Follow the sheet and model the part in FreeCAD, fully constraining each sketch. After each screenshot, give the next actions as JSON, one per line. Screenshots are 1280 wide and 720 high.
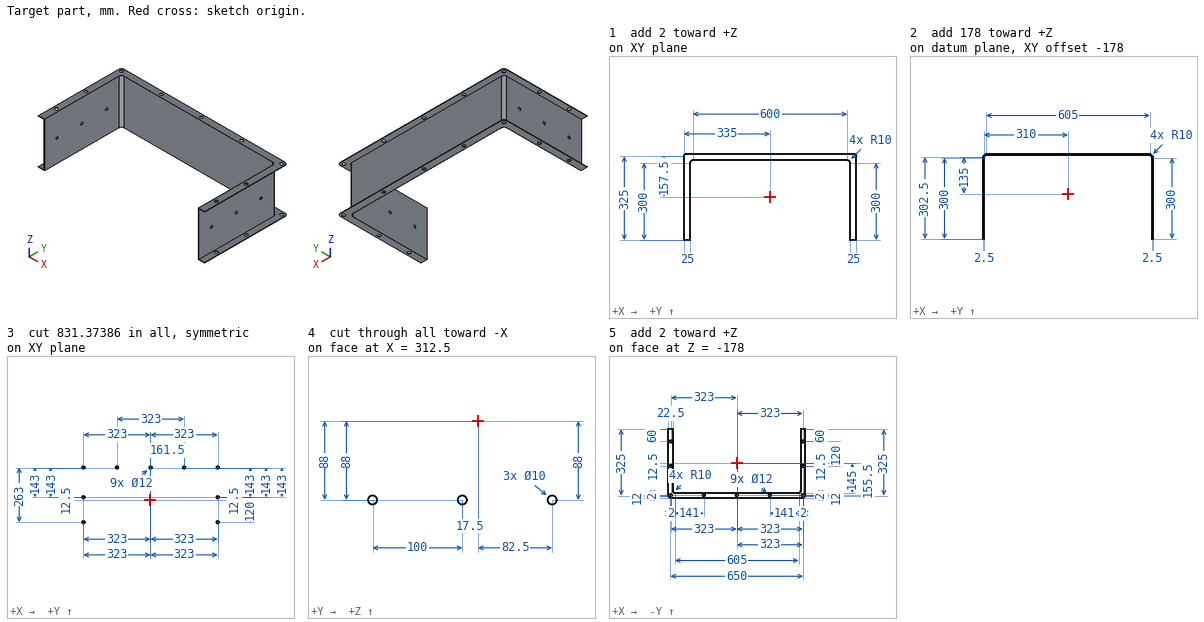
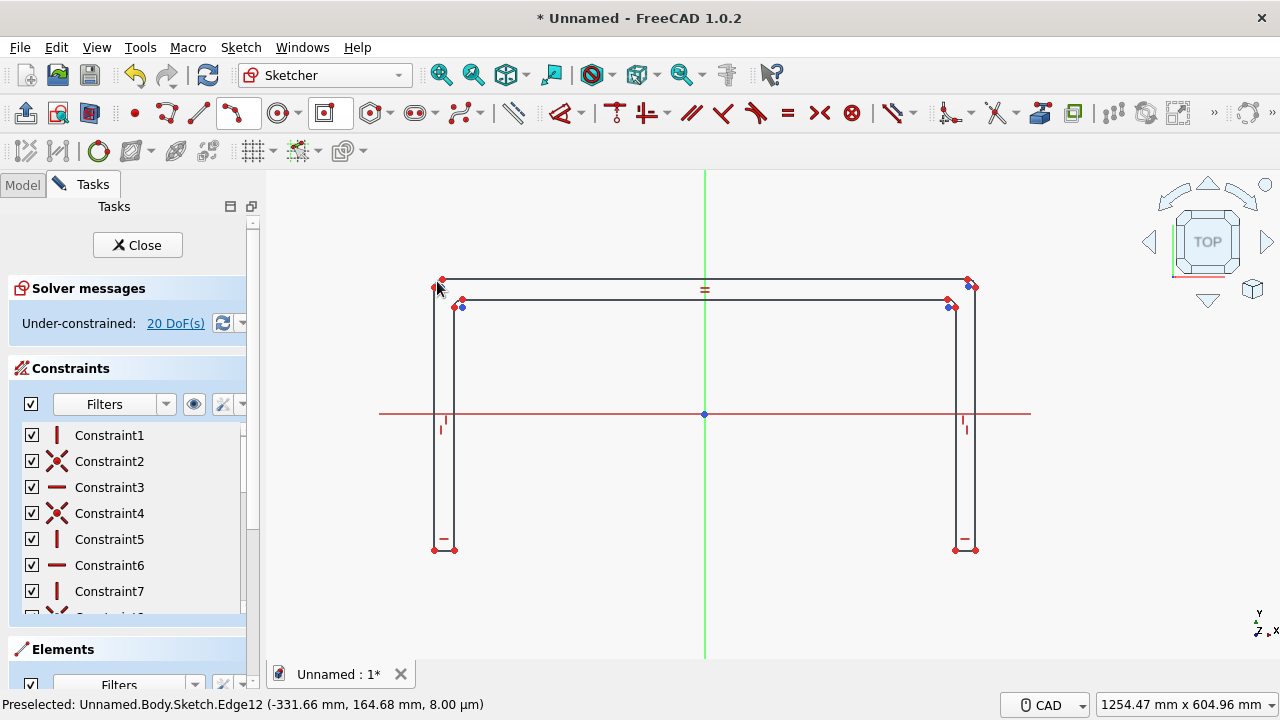
{"action": "left_click", "coordinate": [434, 367]}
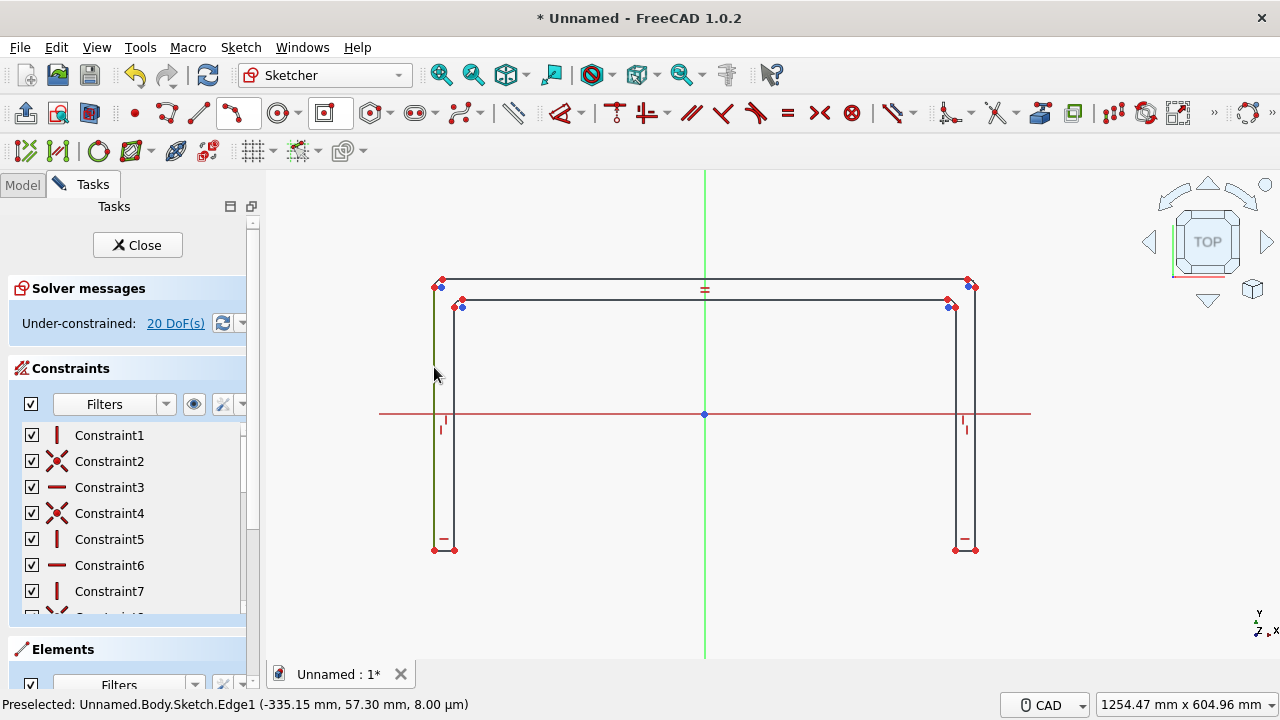
{"action": "scroll", "coordinate": [436, 282], "scroll_direction": "up", "scroll_amount": 4}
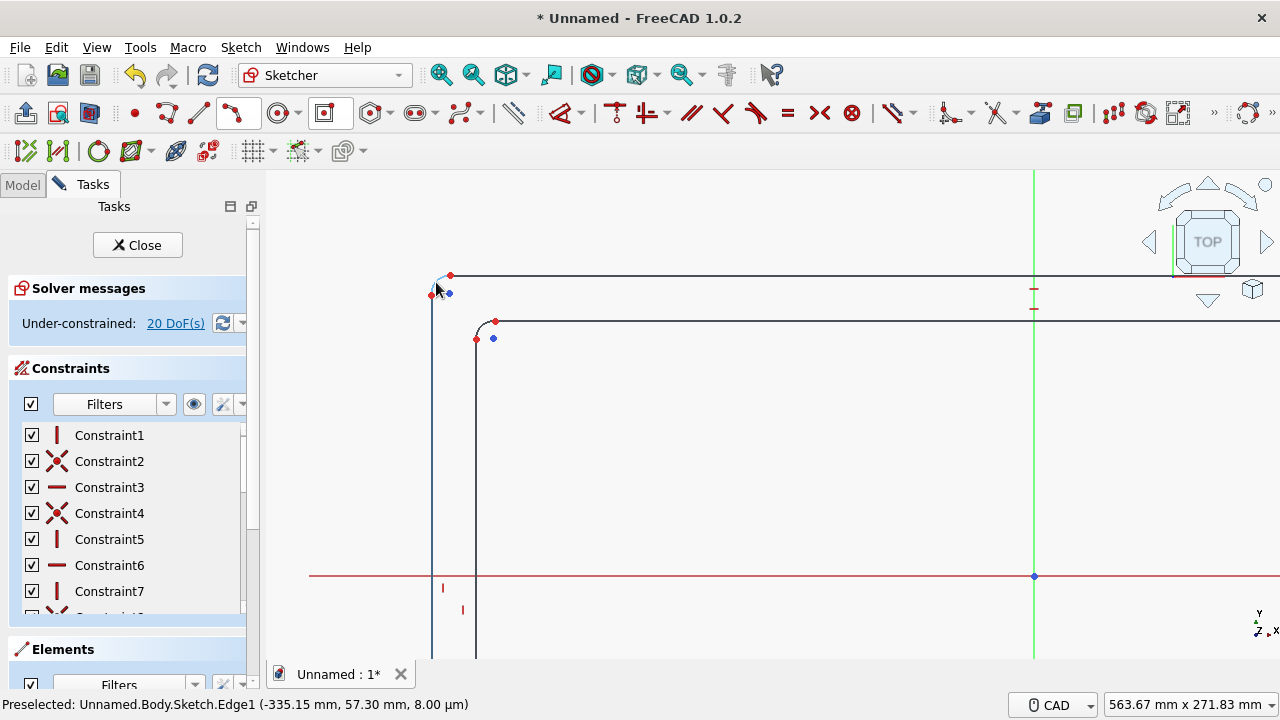
{"action": "left_click", "coordinate": [436, 281]}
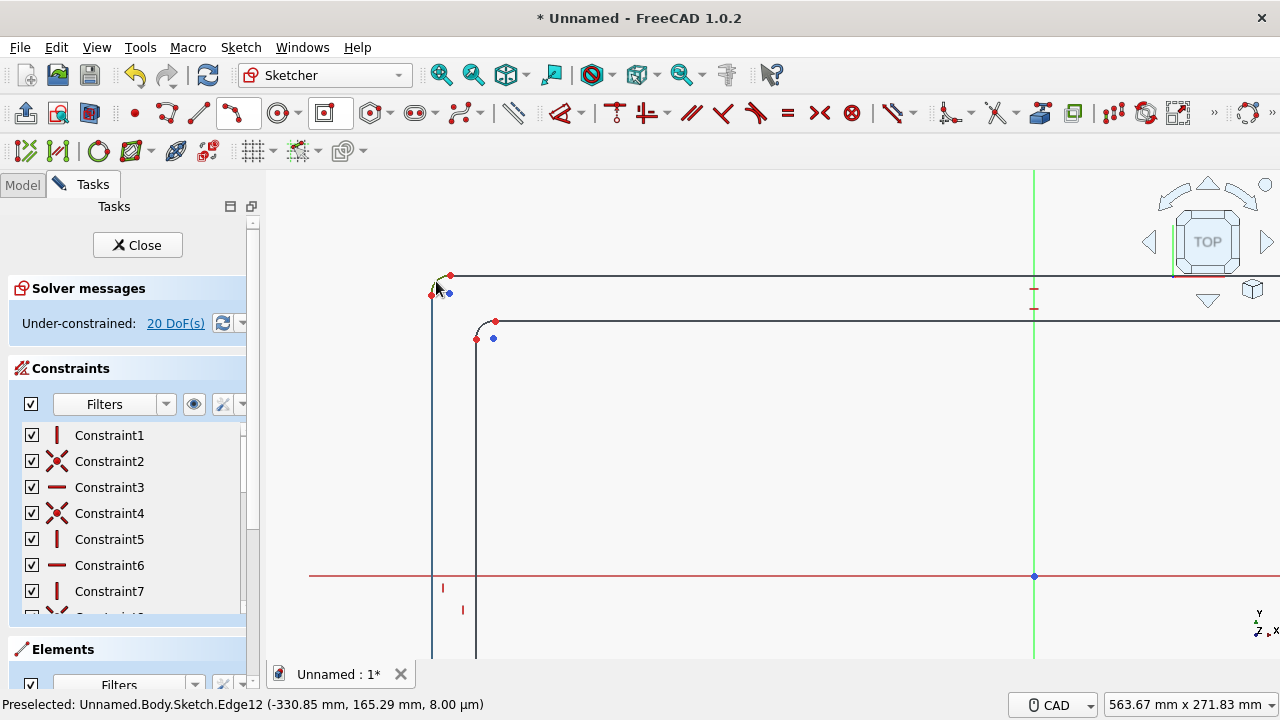
{"action": "left_click", "coordinate": [756, 114]}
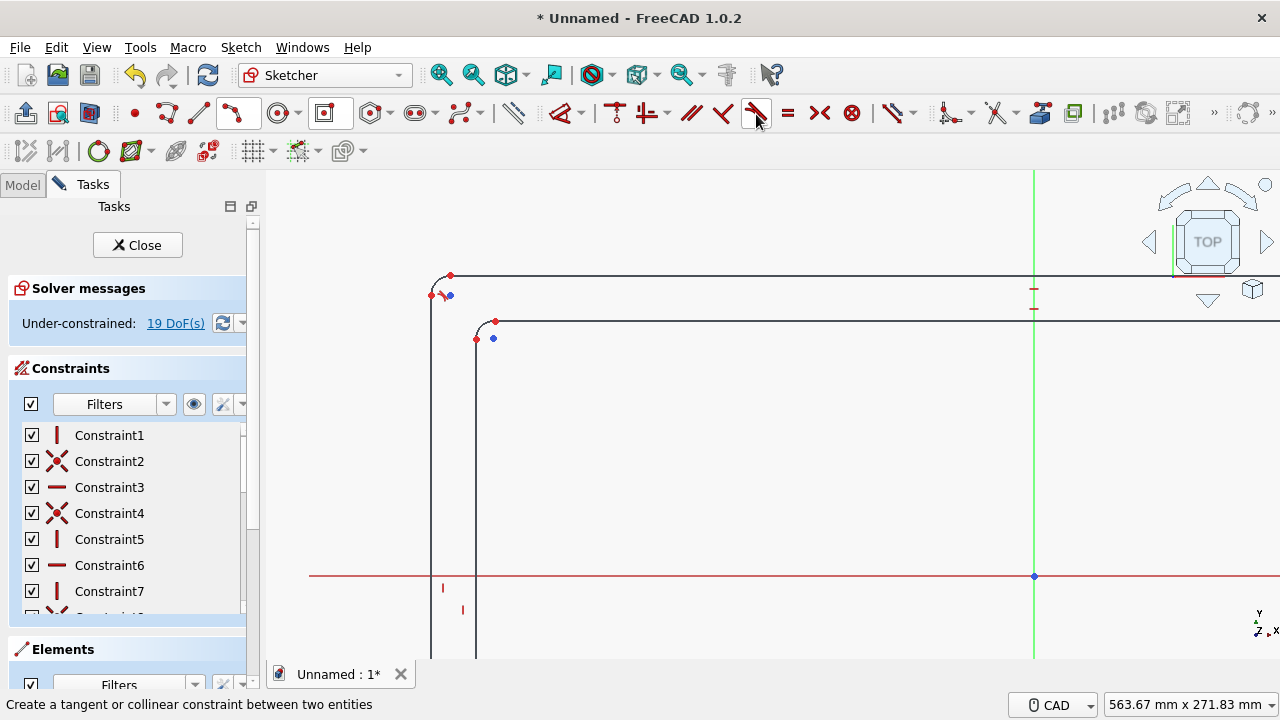
{"action": "left_click", "coordinate": [476, 502]}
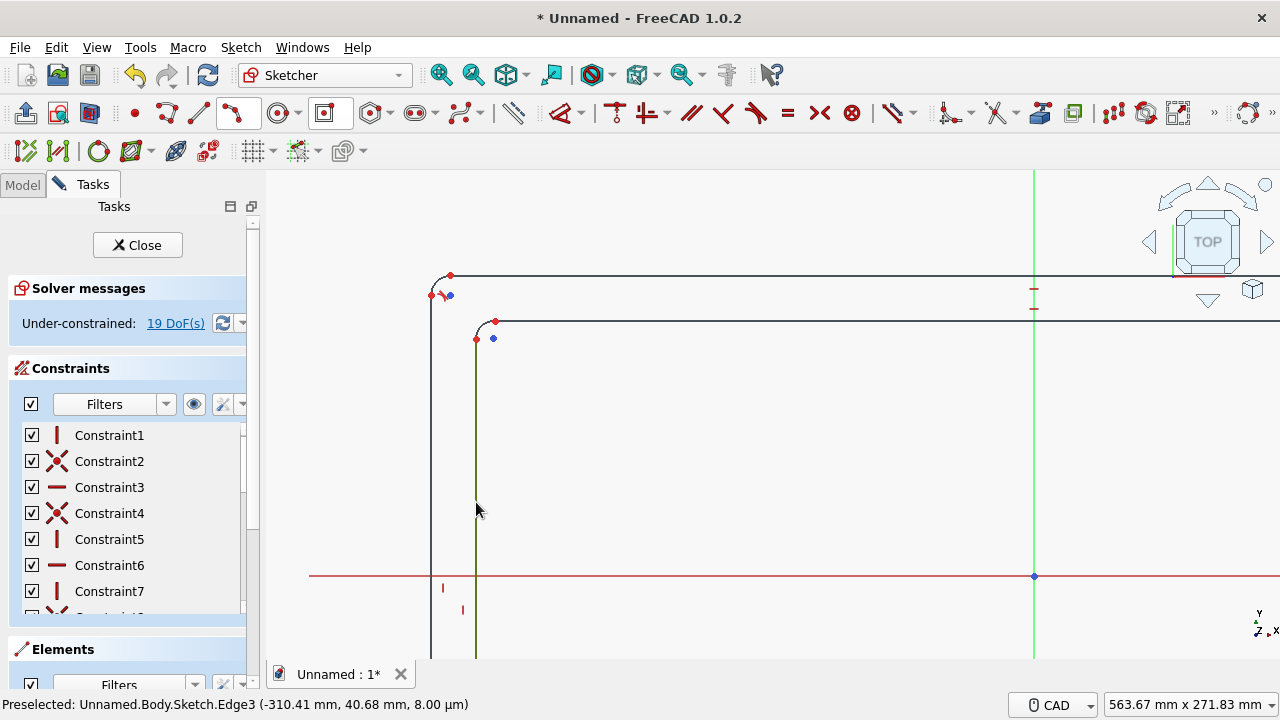
{"action": "left_click", "coordinate": [482, 326]}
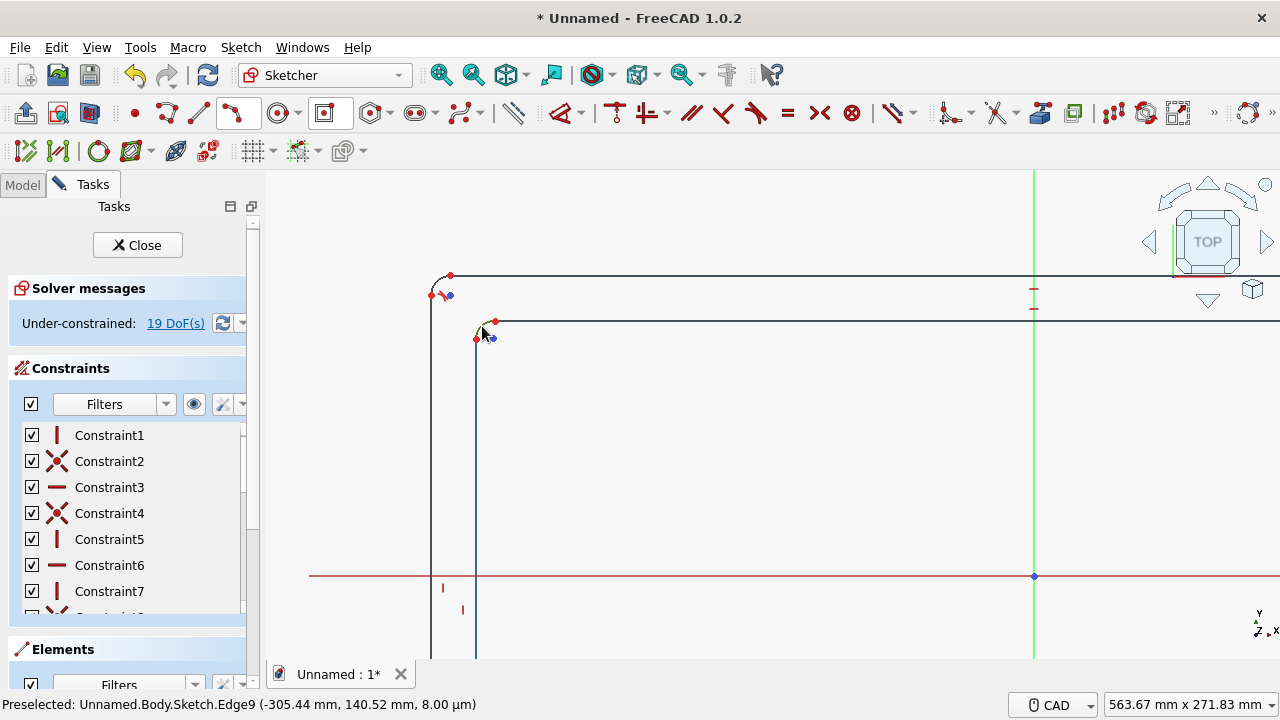
{"action": "left_click", "coordinate": [756, 114]}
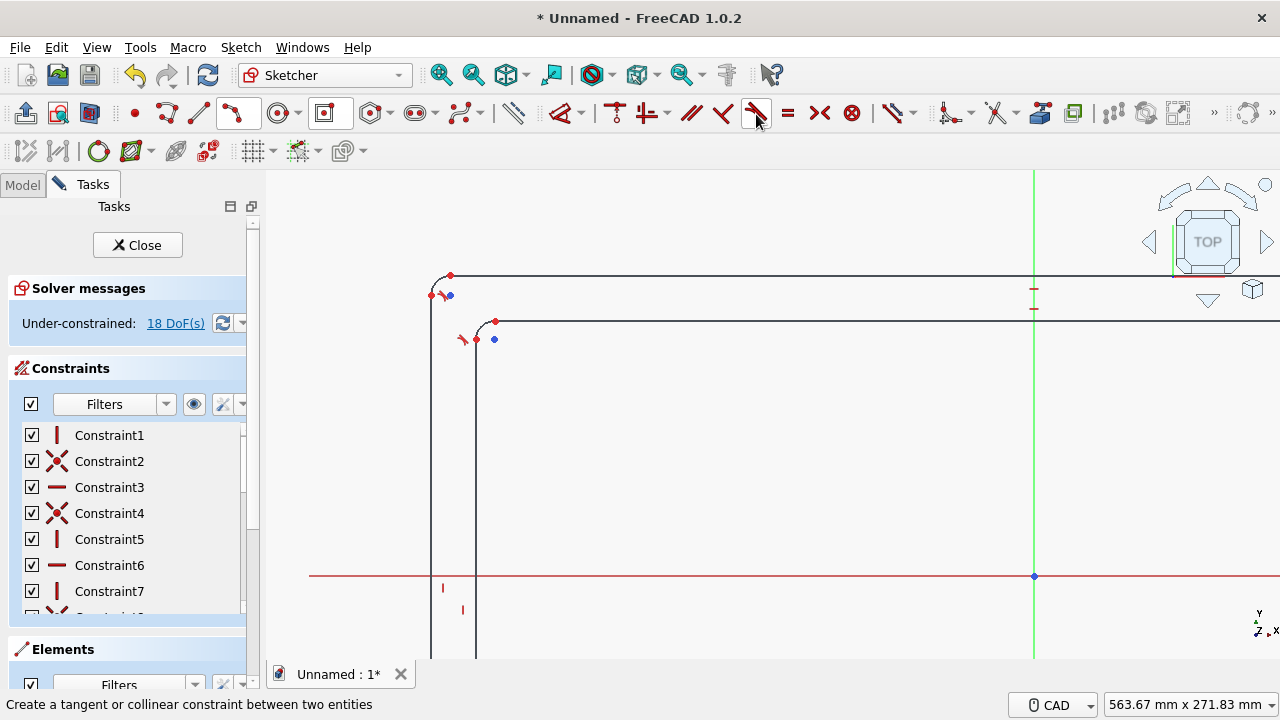
{"action": "left_click", "coordinate": [819, 321]}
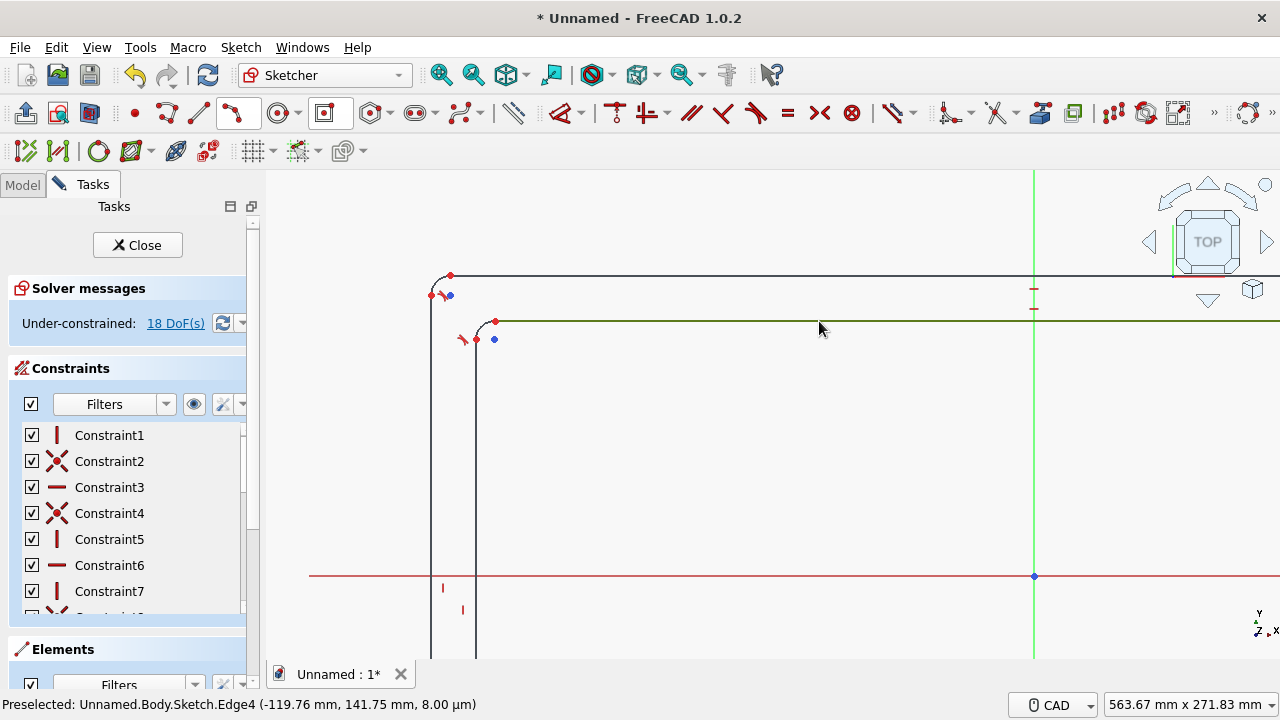
{"action": "left_click", "coordinate": [482, 326]}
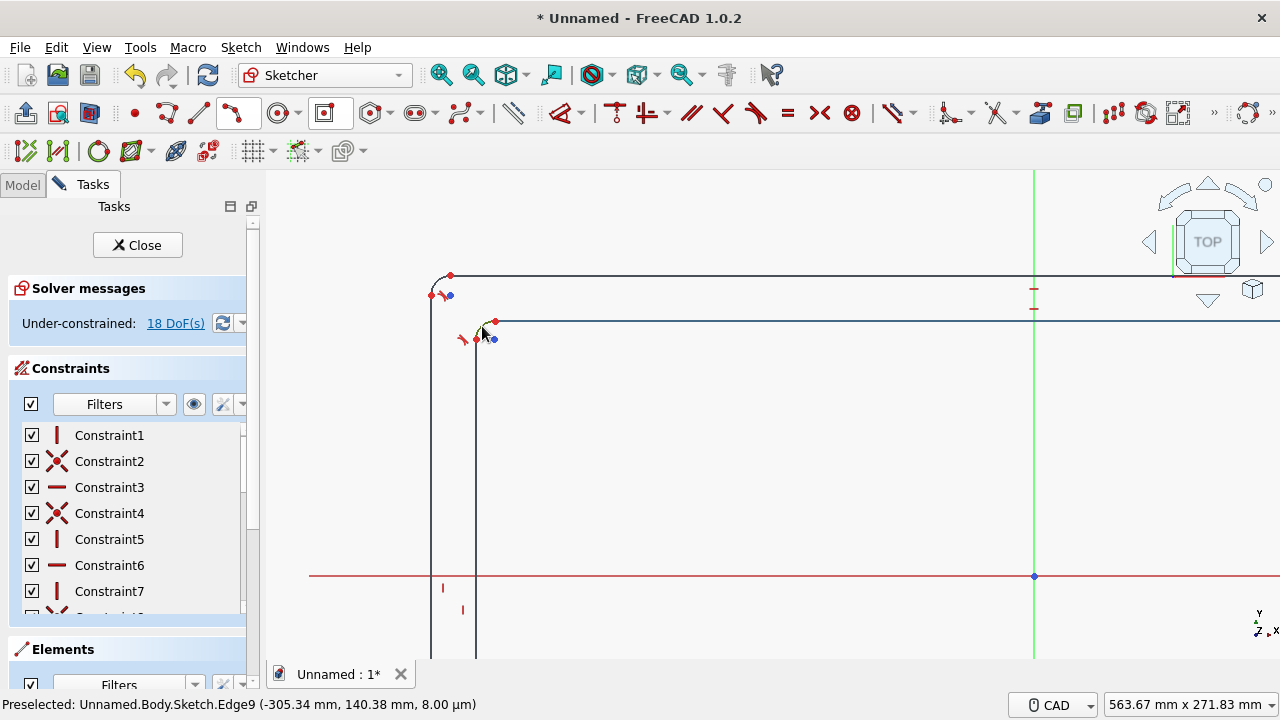
{"action": "key", "text": "t"}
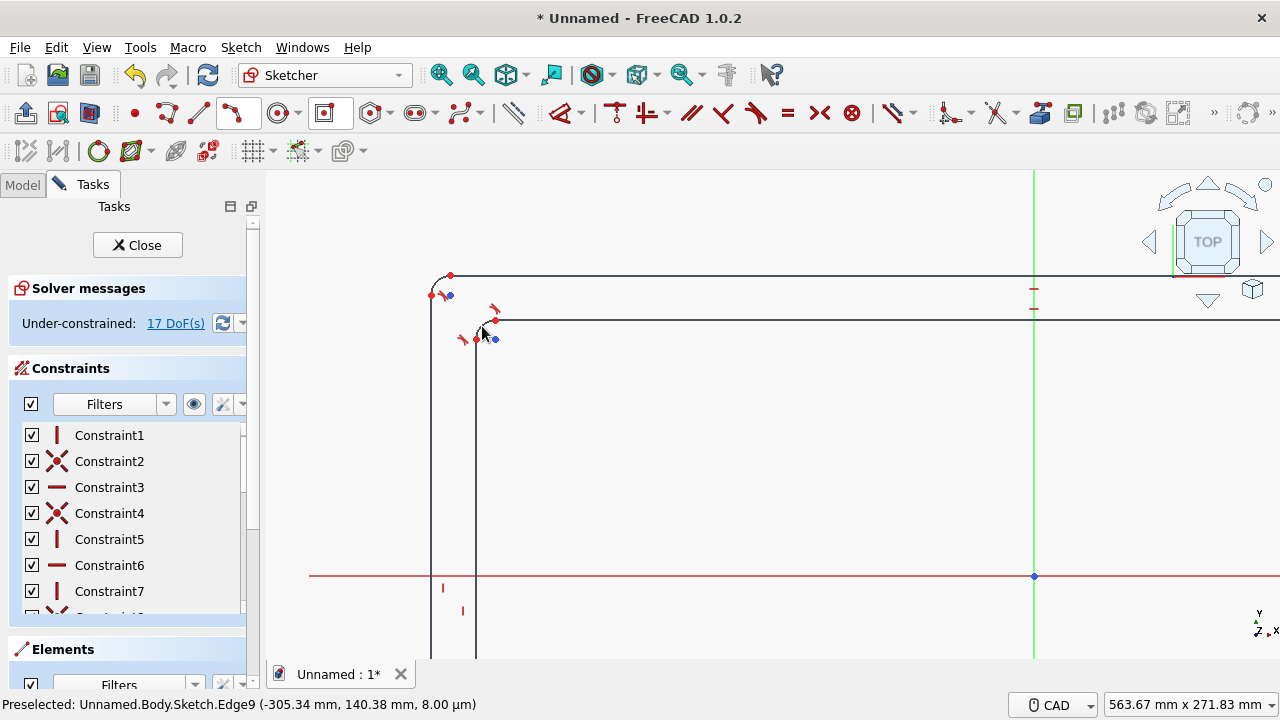
{"action": "left_click", "coordinate": [819, 320]}